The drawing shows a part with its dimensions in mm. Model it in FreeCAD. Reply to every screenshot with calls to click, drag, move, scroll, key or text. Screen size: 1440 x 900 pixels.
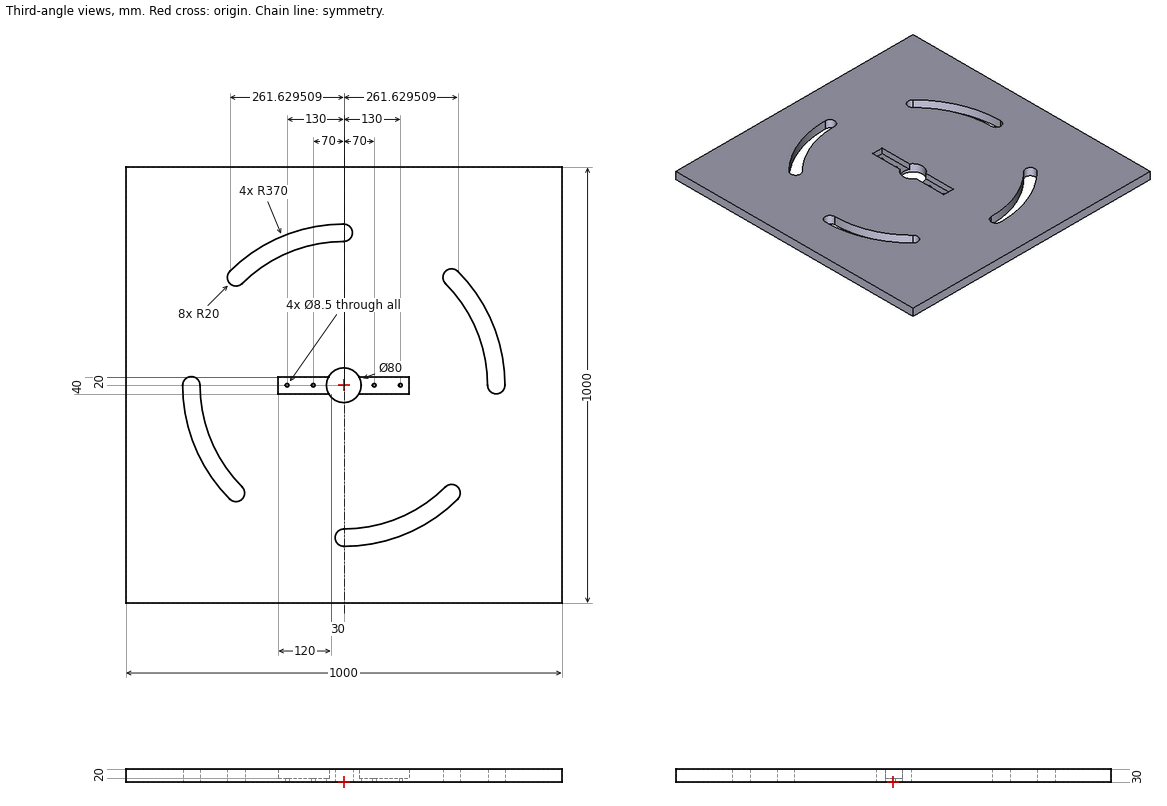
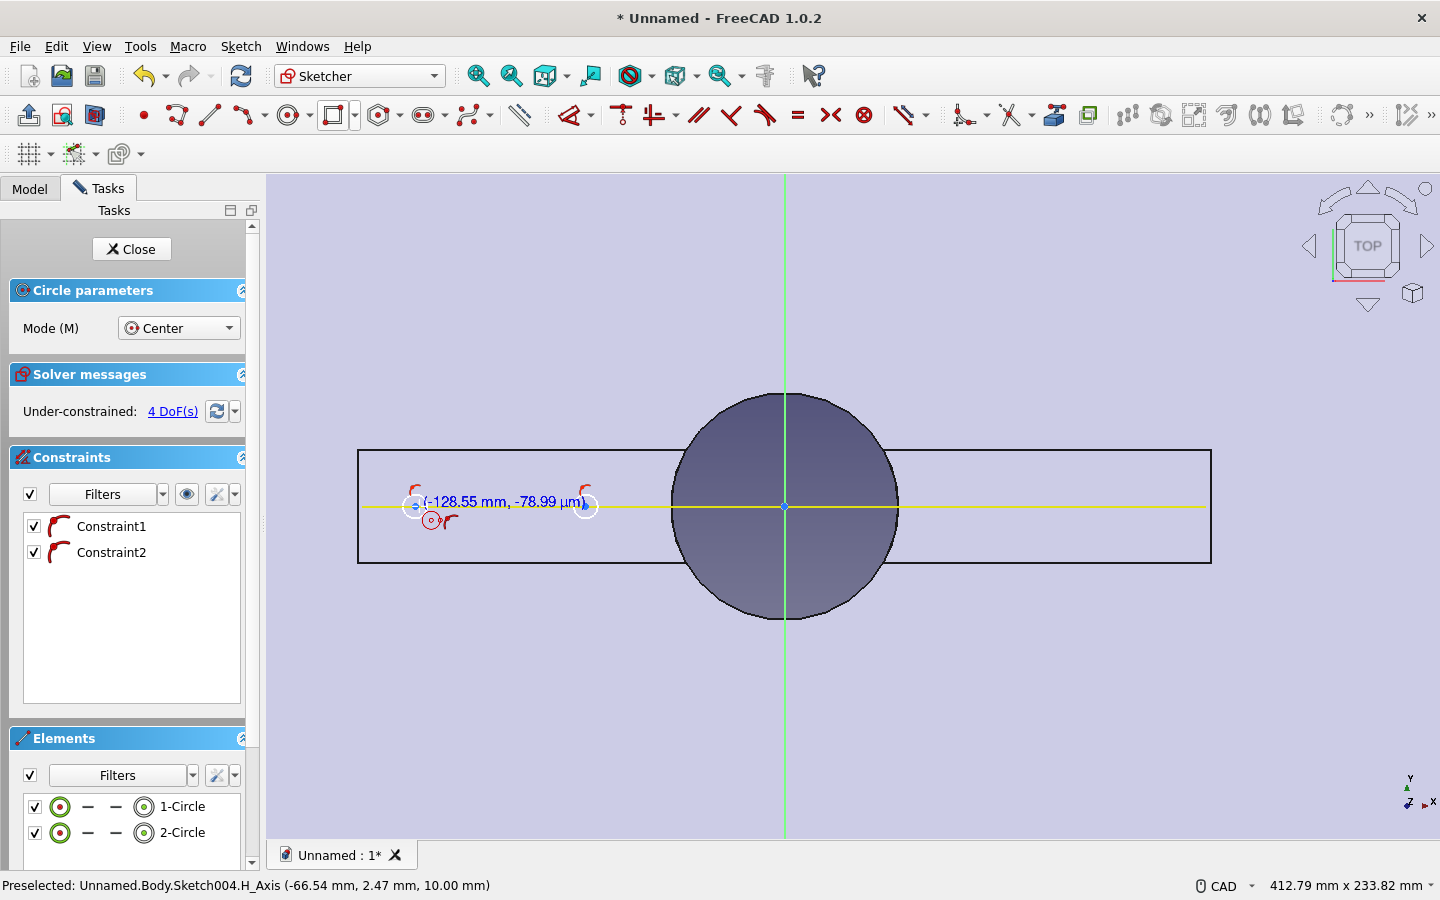
scroll(984, 506, up, 4)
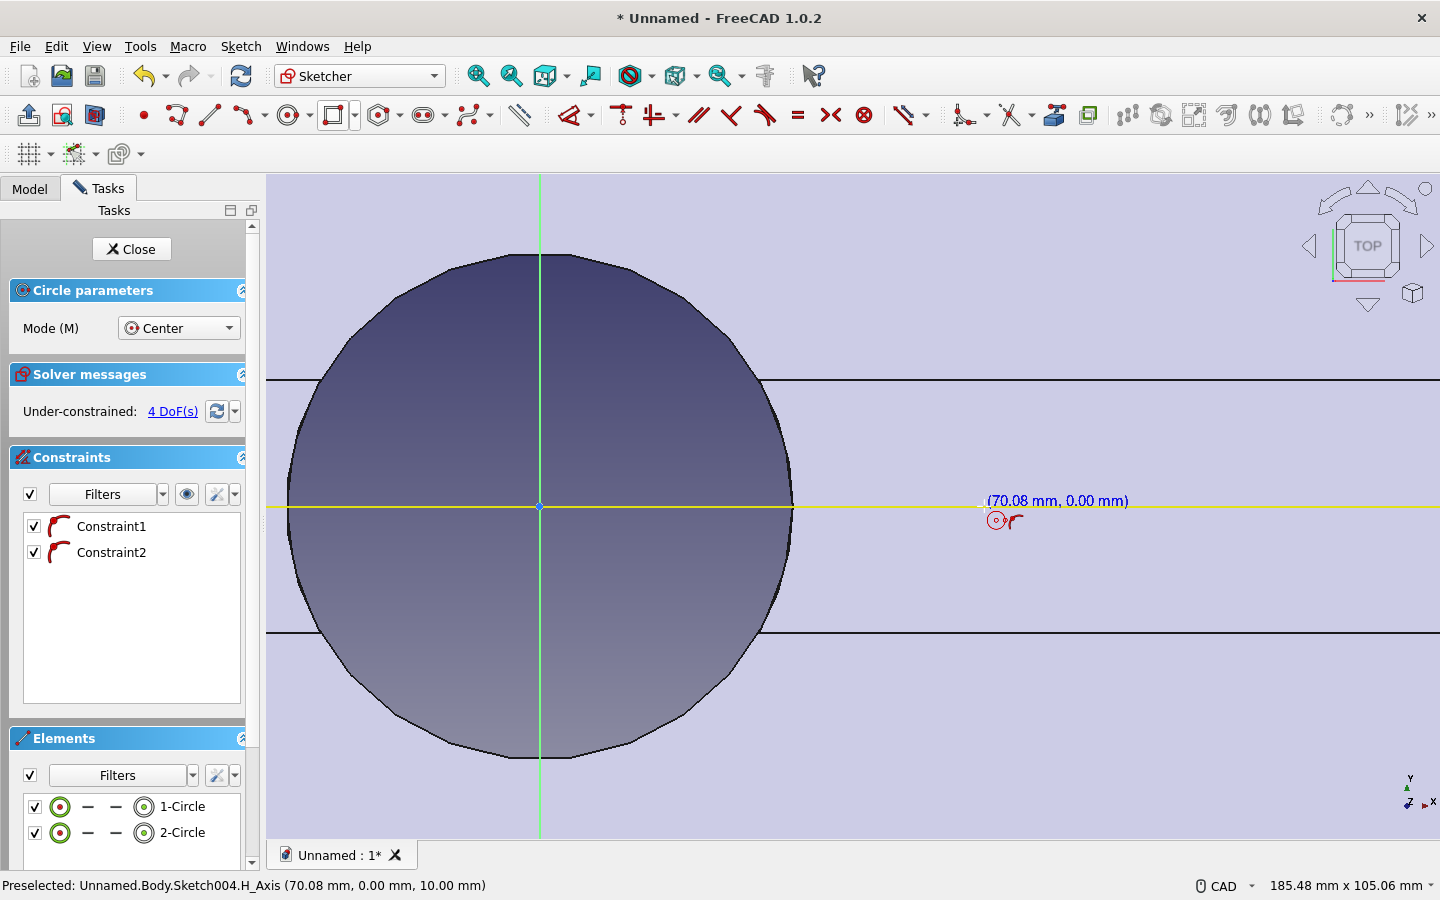
click(983, 506)
click(1002, 487)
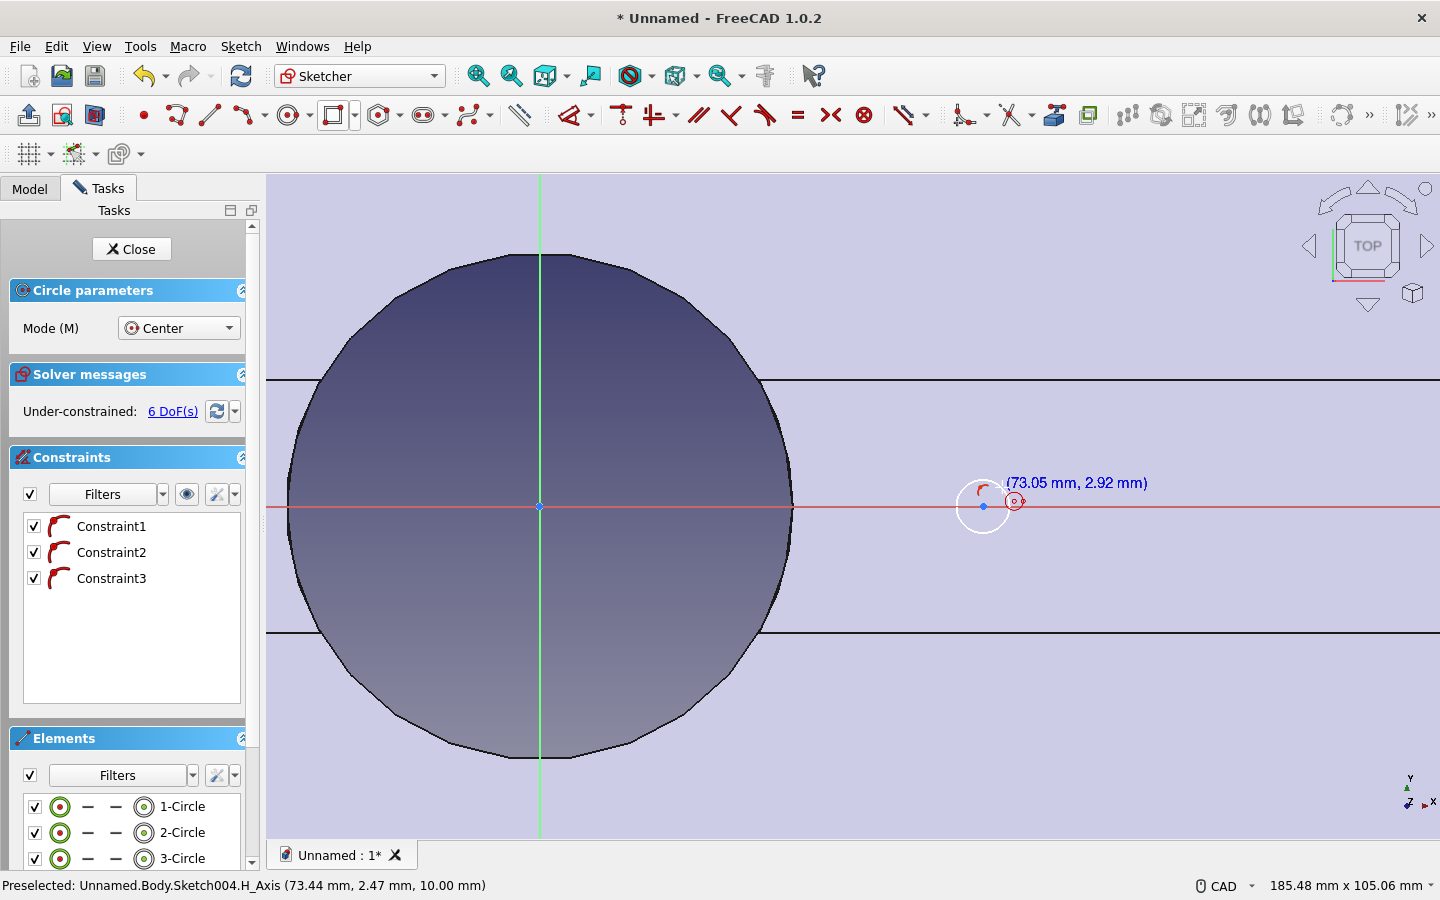
scroll(984, 506, down, 4)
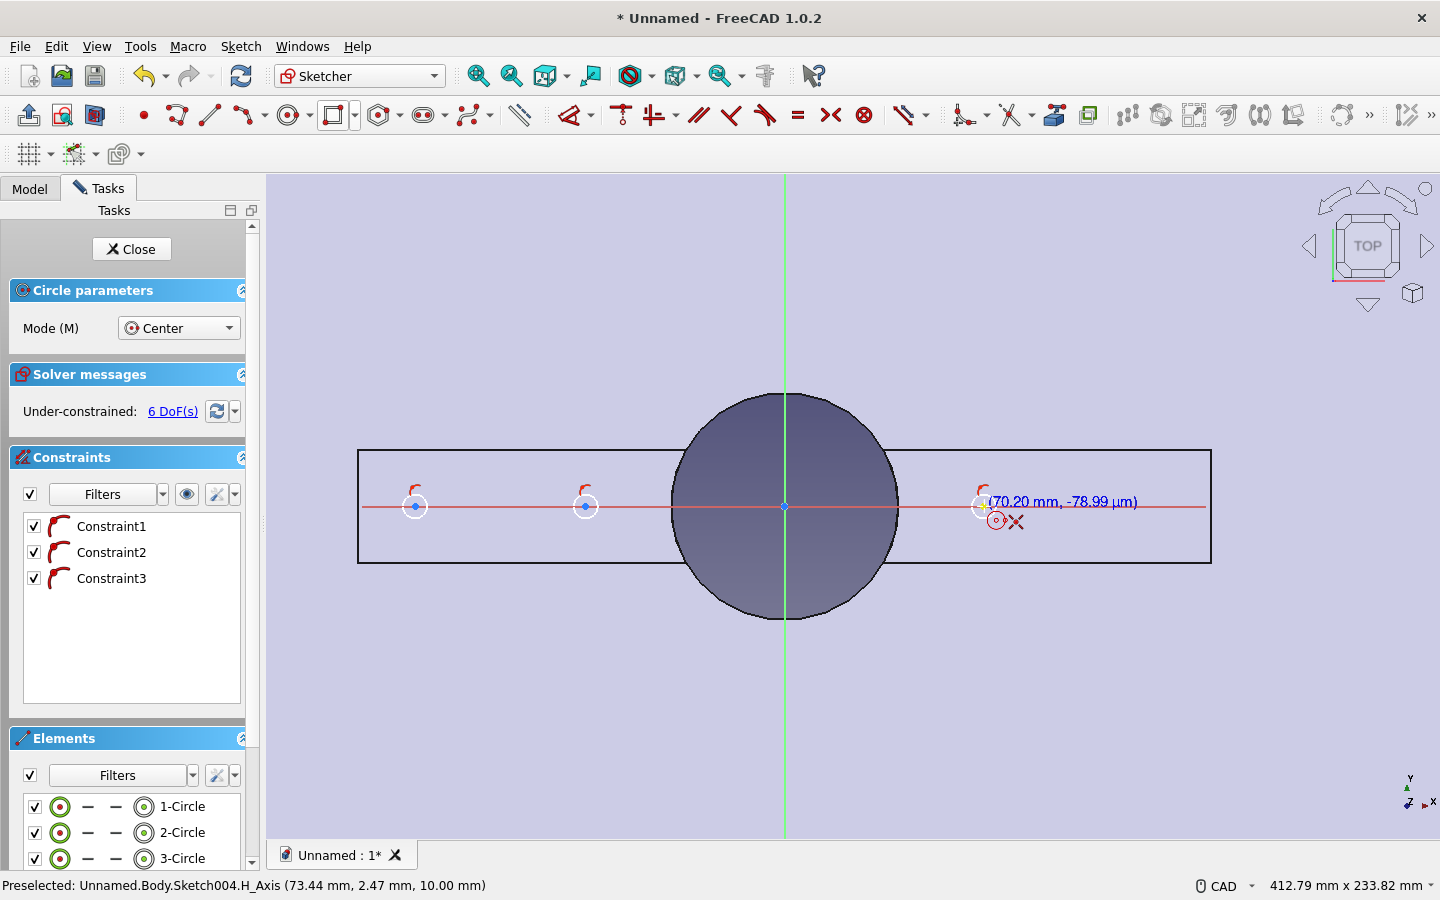
scroll(1154, 506, up, 4)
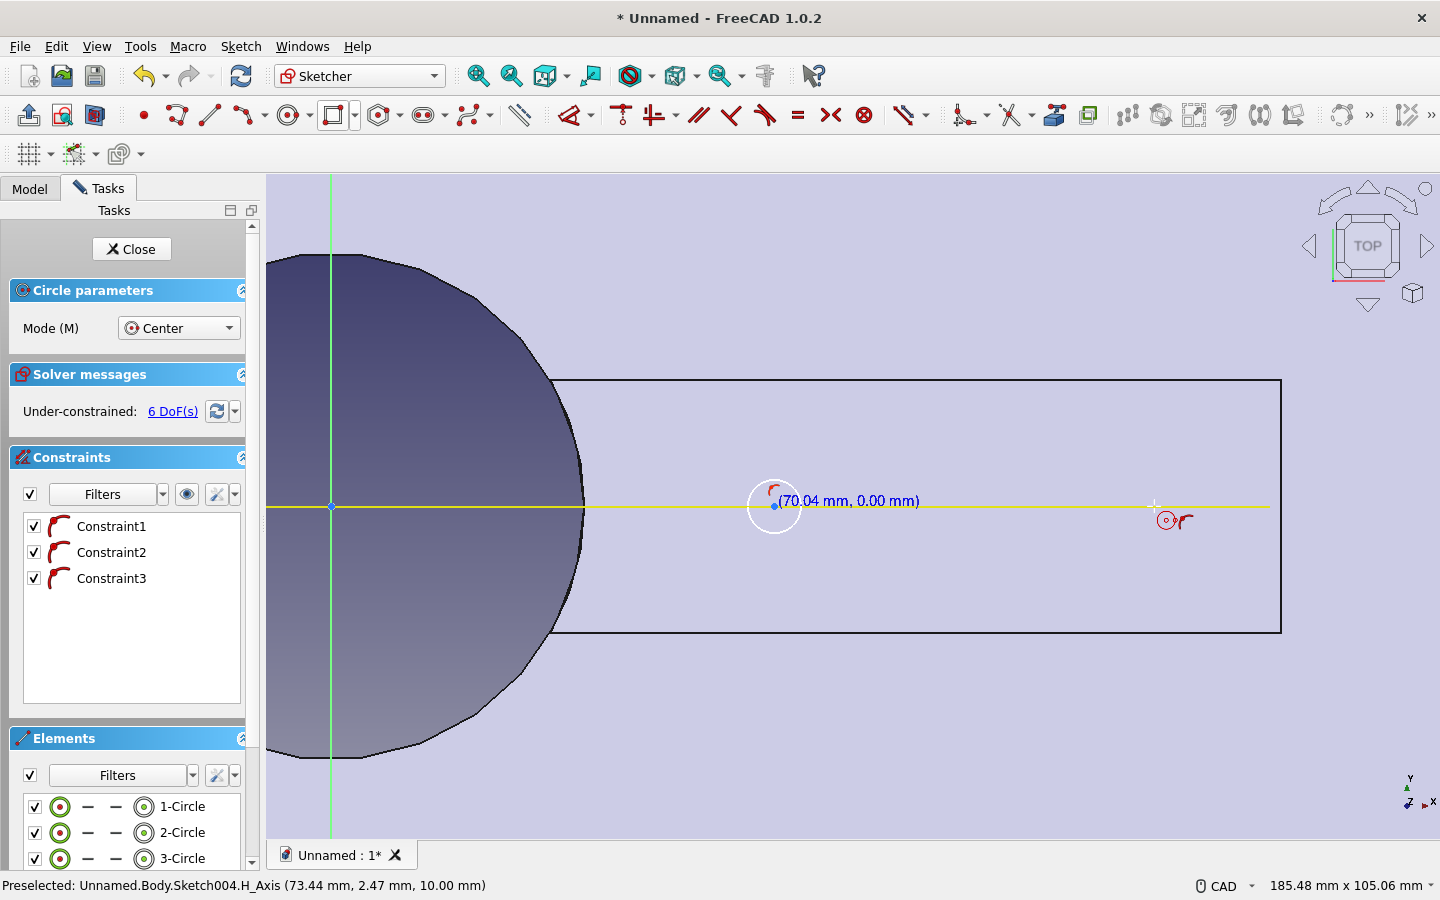
click(1154, 506)
click(1173, 487)
key(Escape)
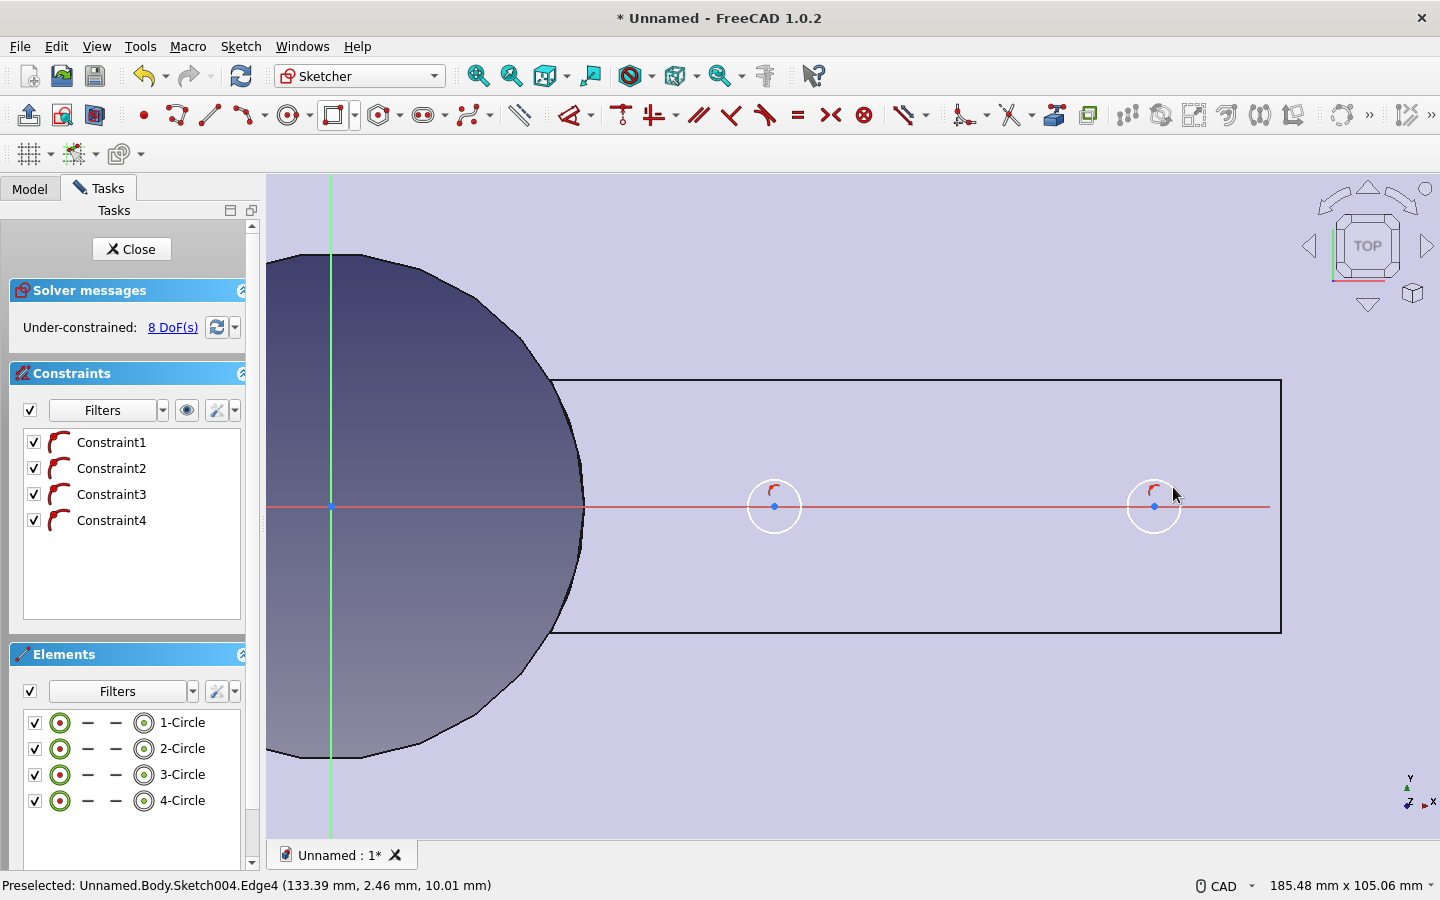
scroll(1154, 506, down, 4)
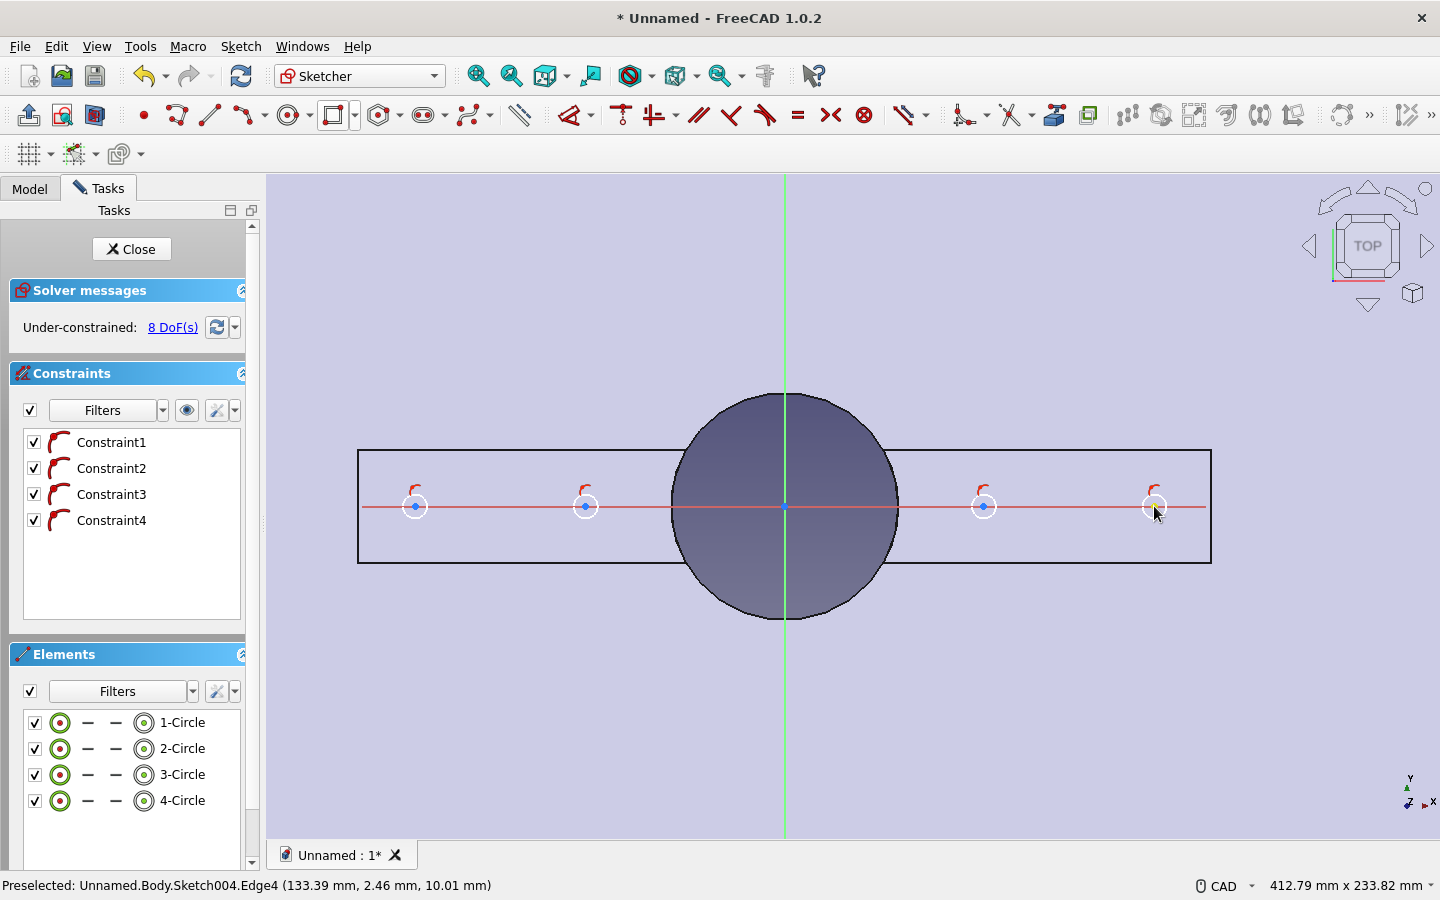
scroll(423, 498, up, 3)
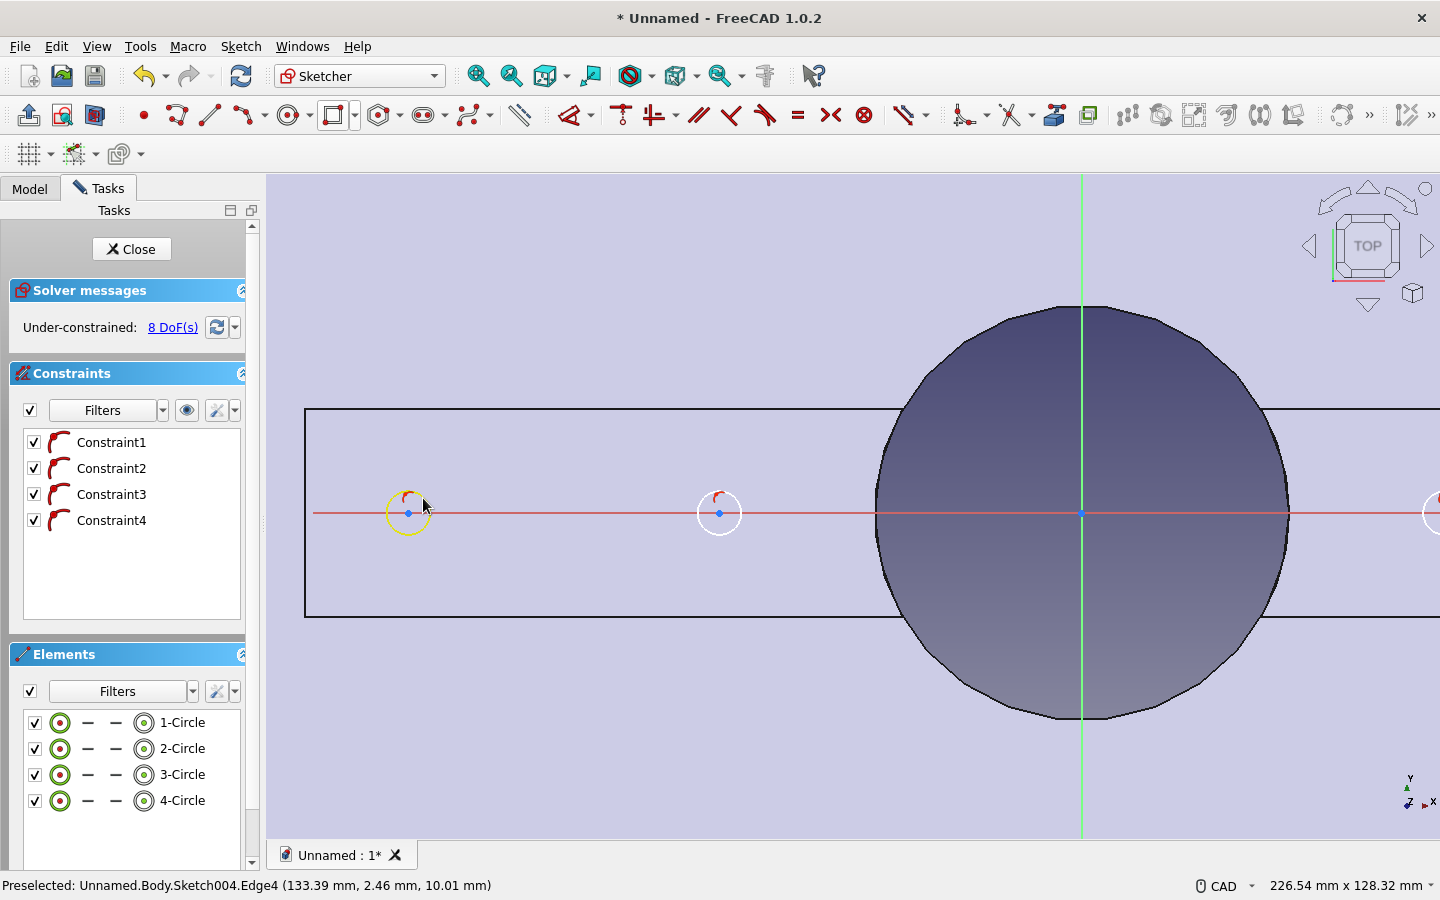
click(424, 498)